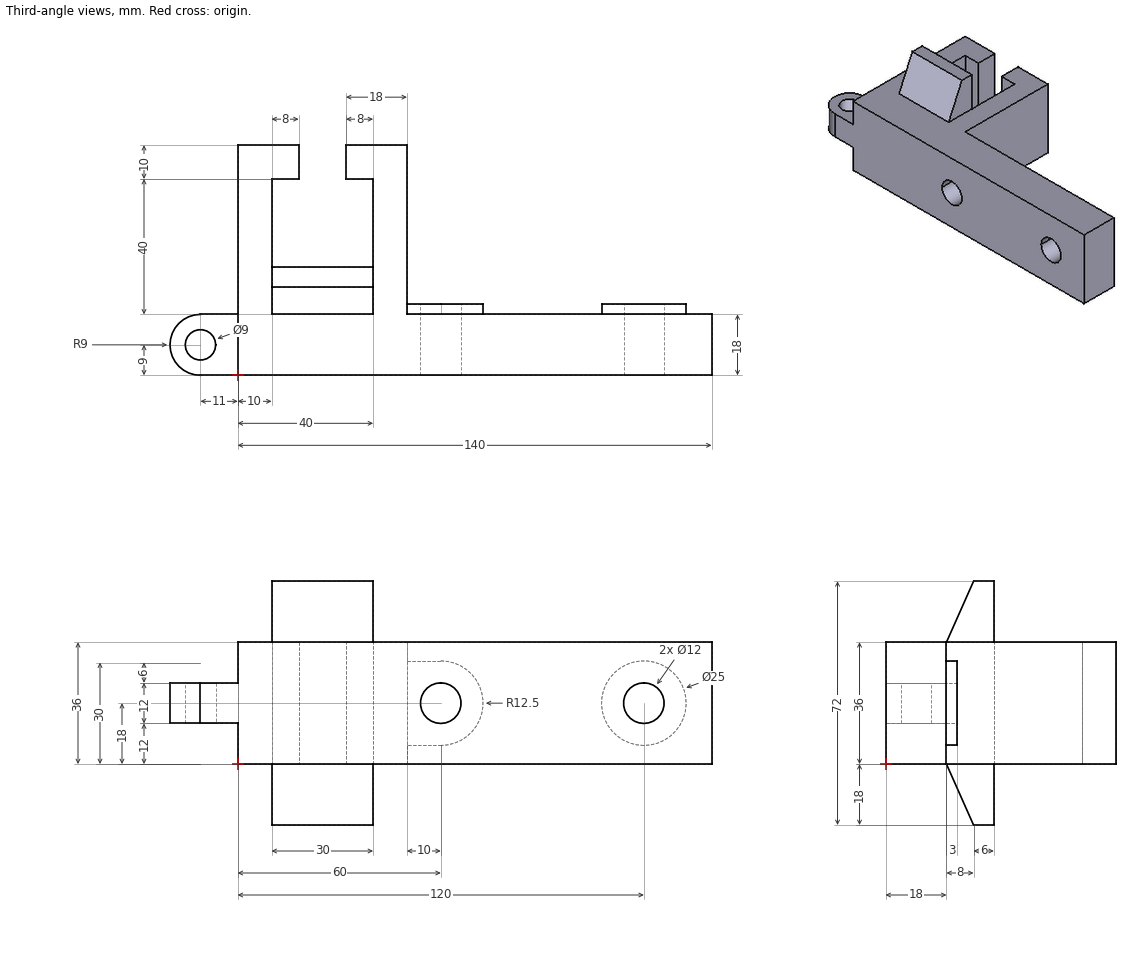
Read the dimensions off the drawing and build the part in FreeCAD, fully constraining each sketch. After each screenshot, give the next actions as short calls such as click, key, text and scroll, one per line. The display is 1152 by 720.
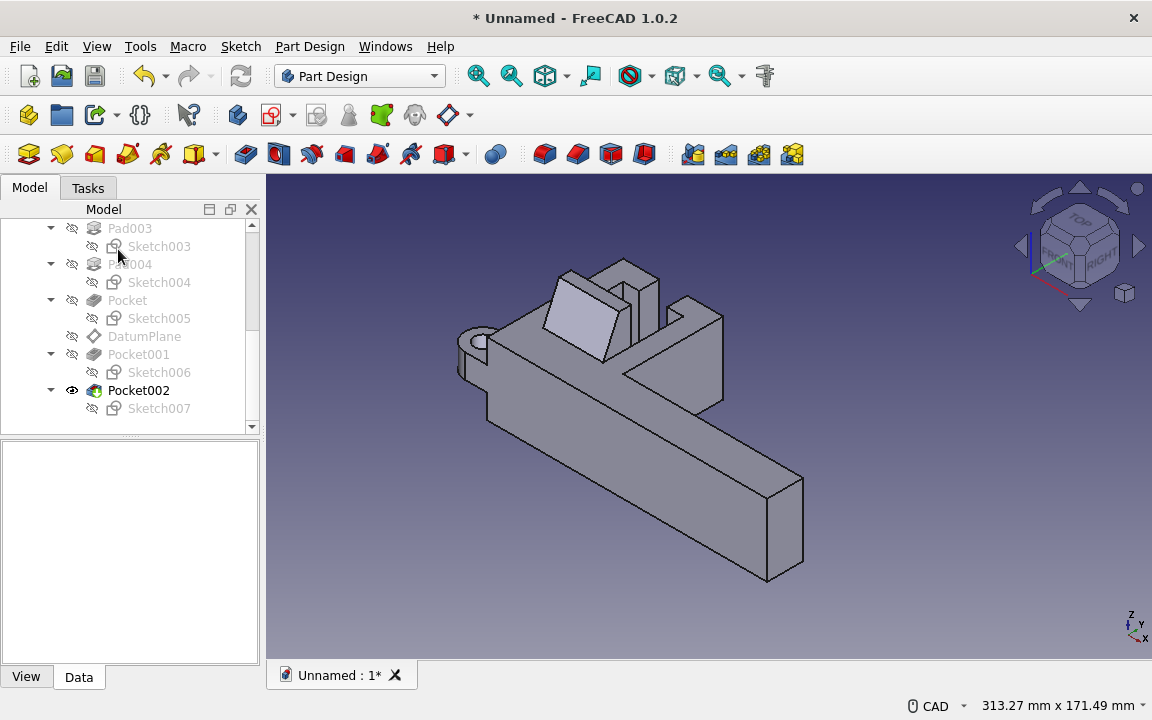
key(4)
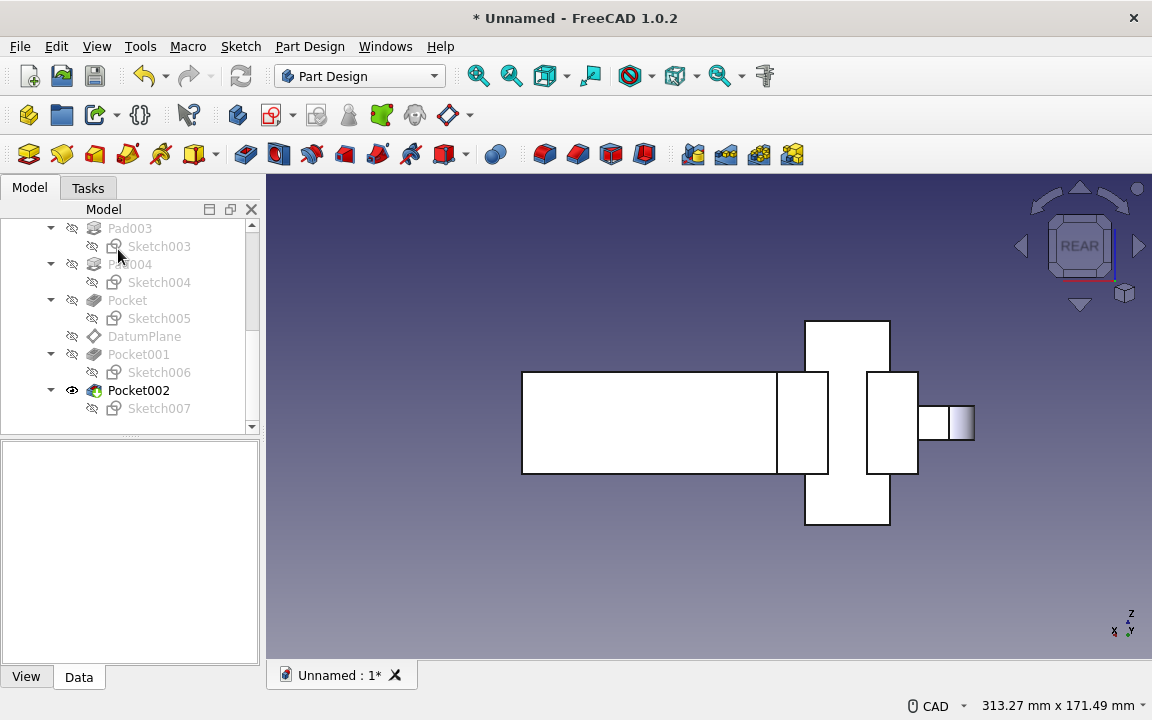
click(577, 422)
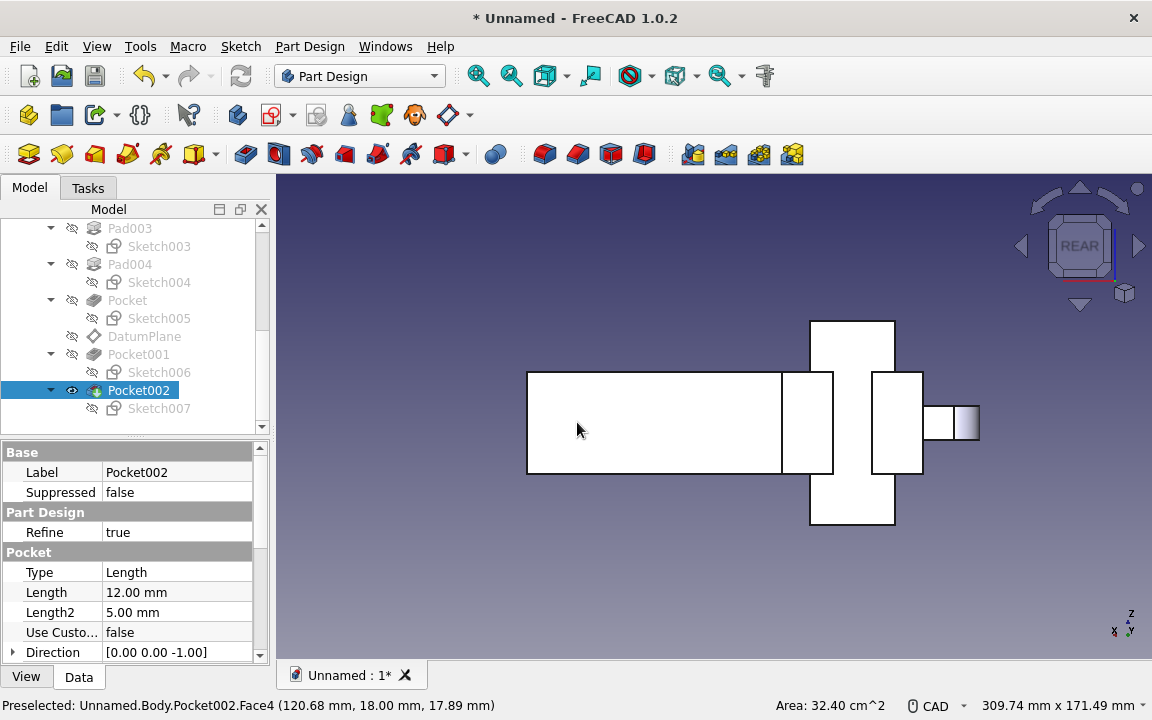
click(270, 116)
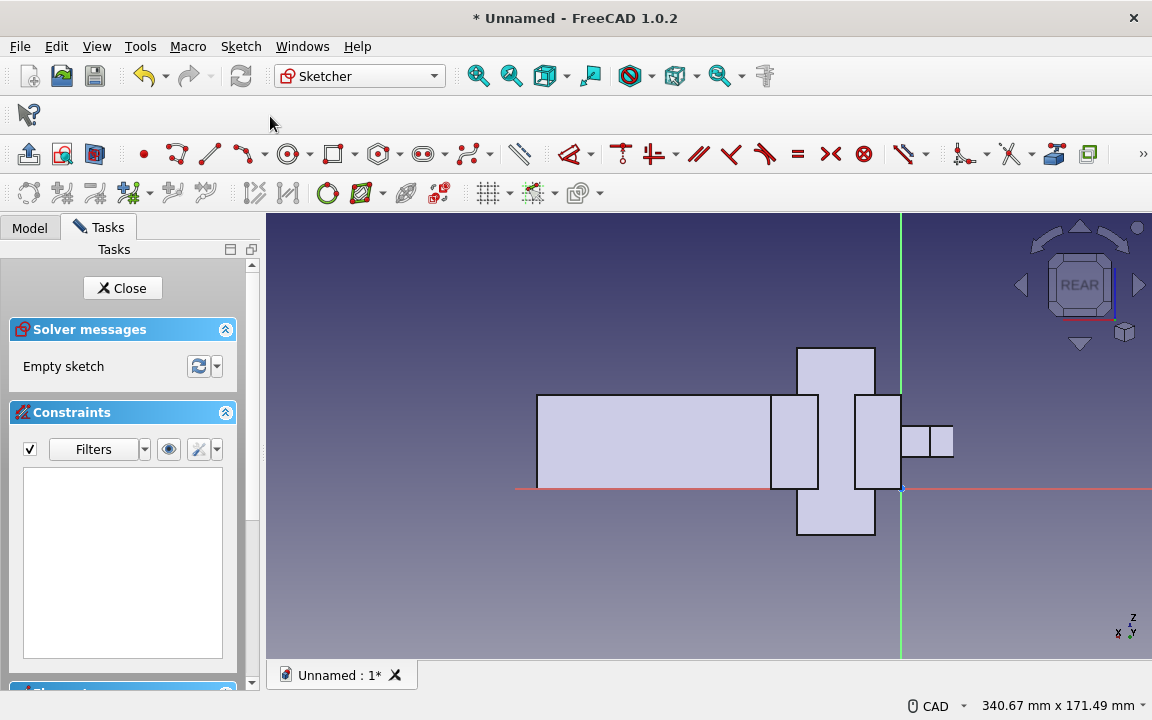
scroll(775, 444, up, 7)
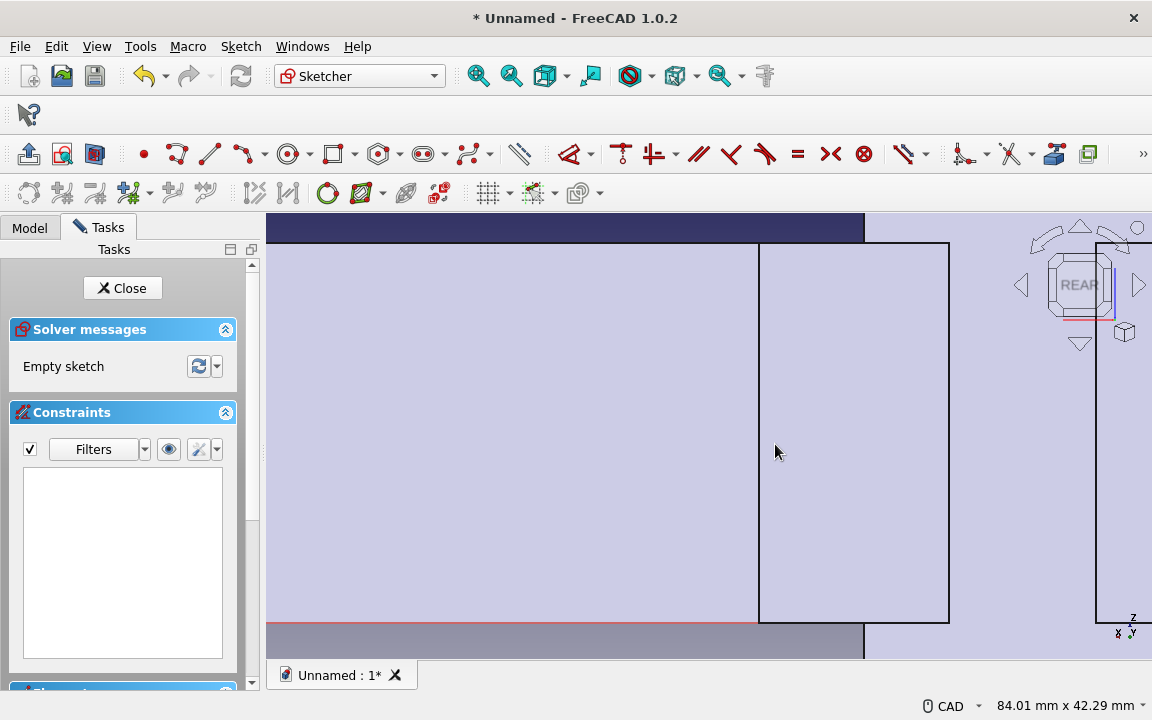
key(g)
key(m)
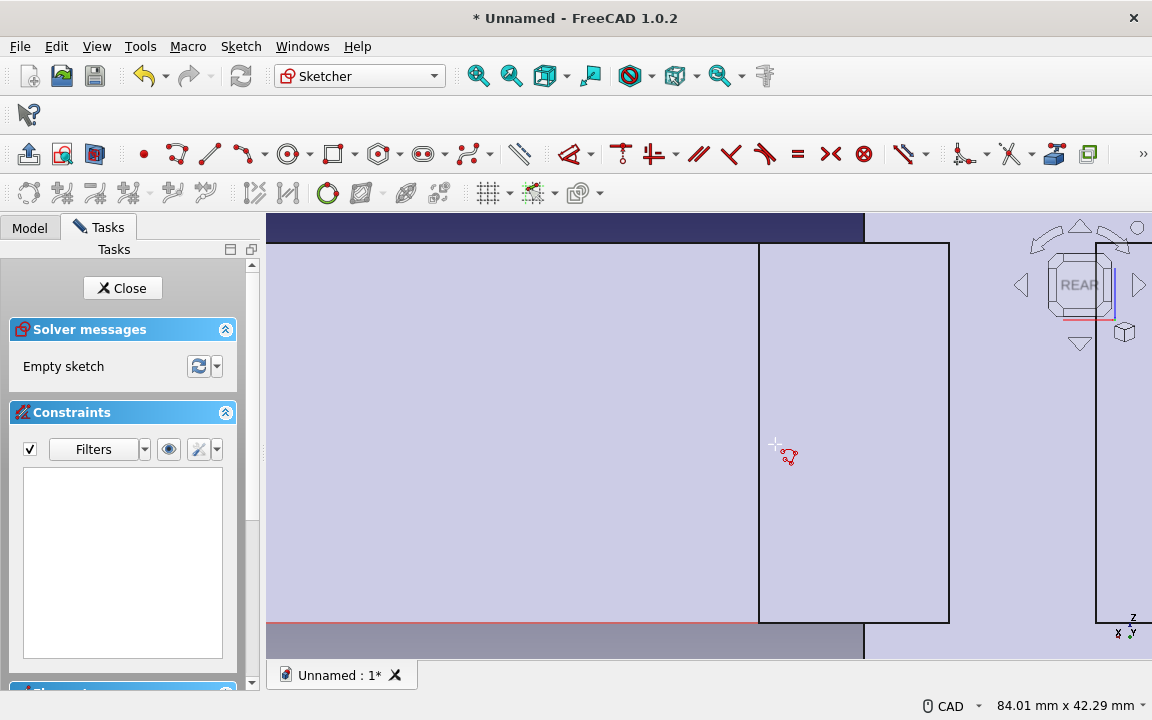
click(653, 565)
click(759, 565)
click(759, 301)
click(653, 301)
right_click(653, 301)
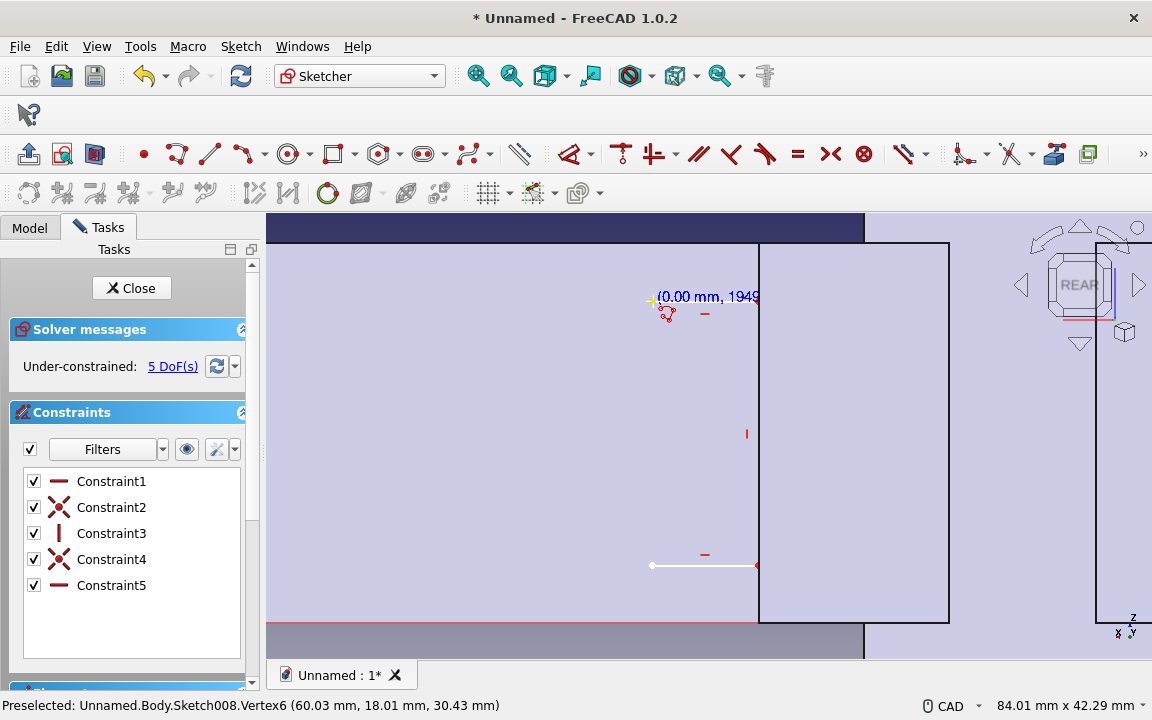
key(g)
key(3)
key(a)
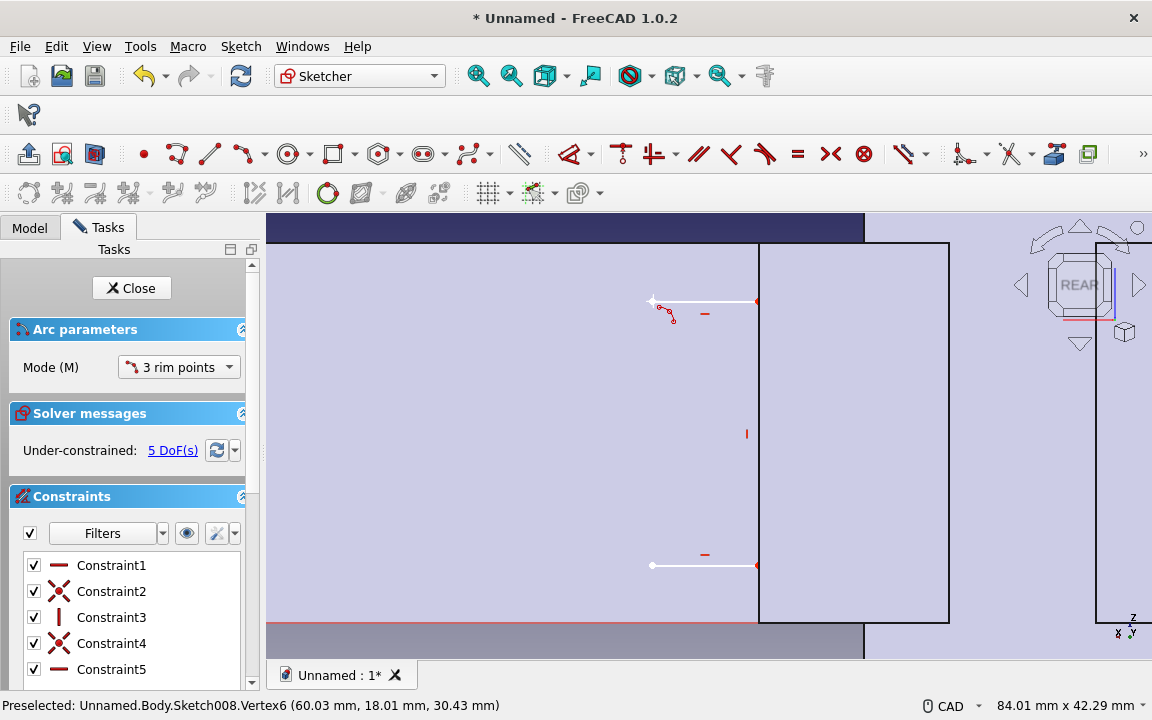
click(653, 302)
click(653, 566)
click(521, 433)
key(Escape)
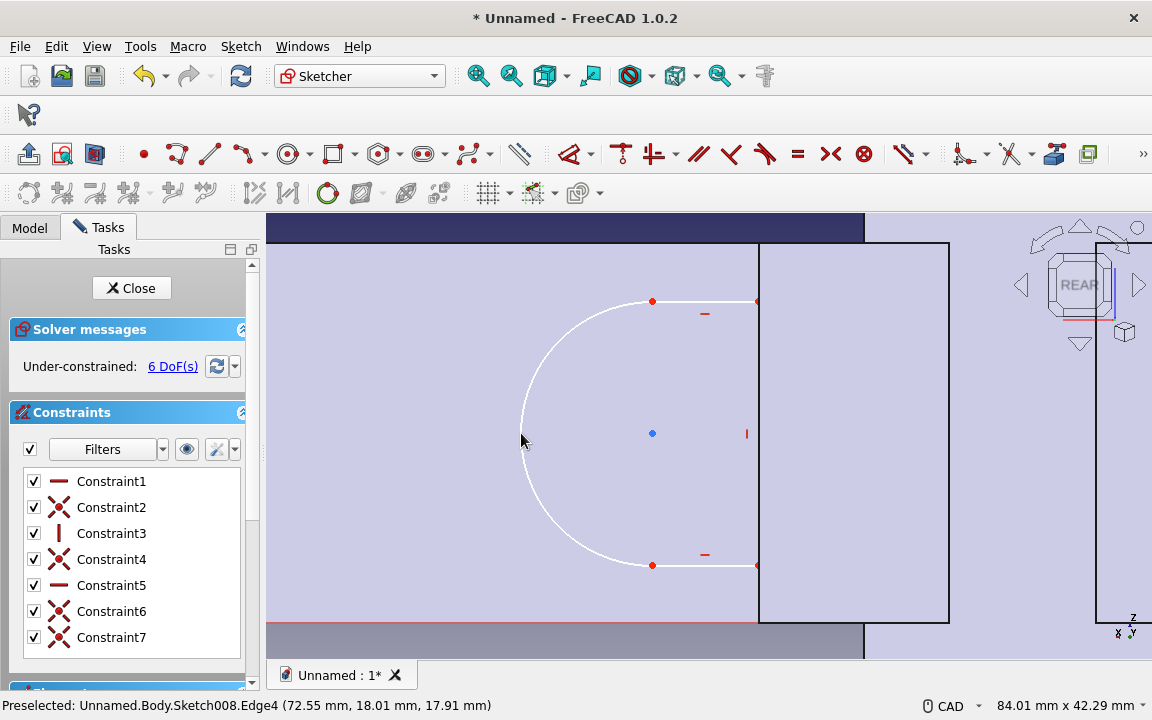
click(685, 566)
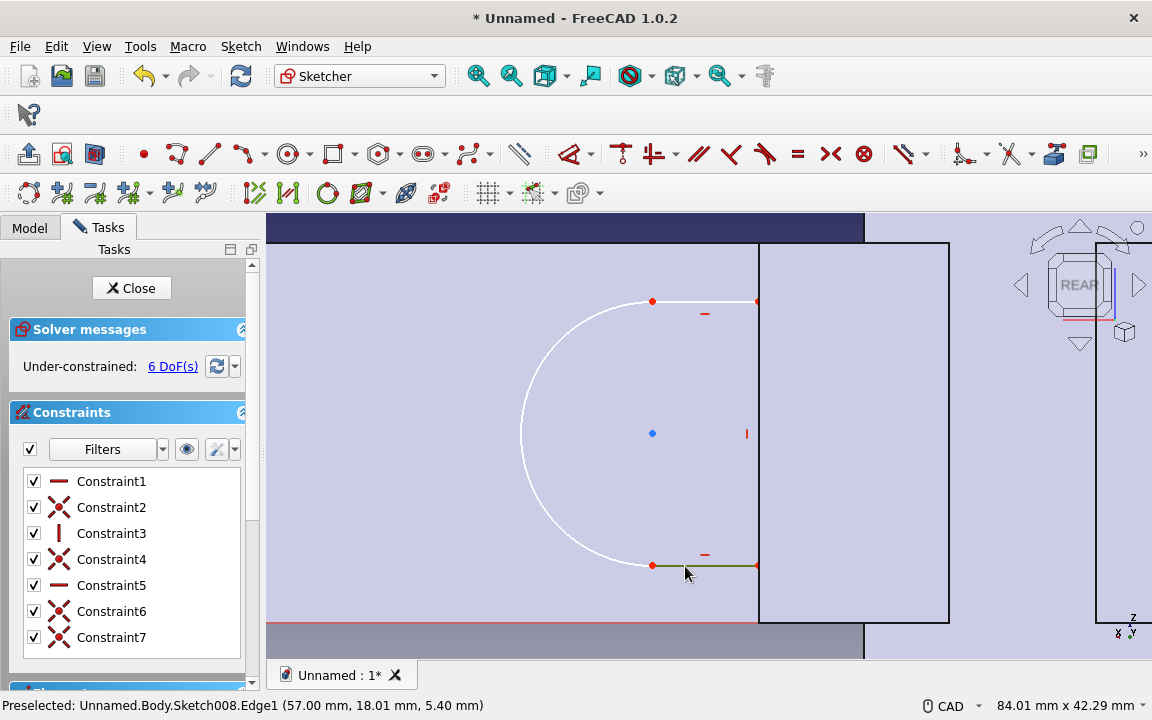
click(546, 356)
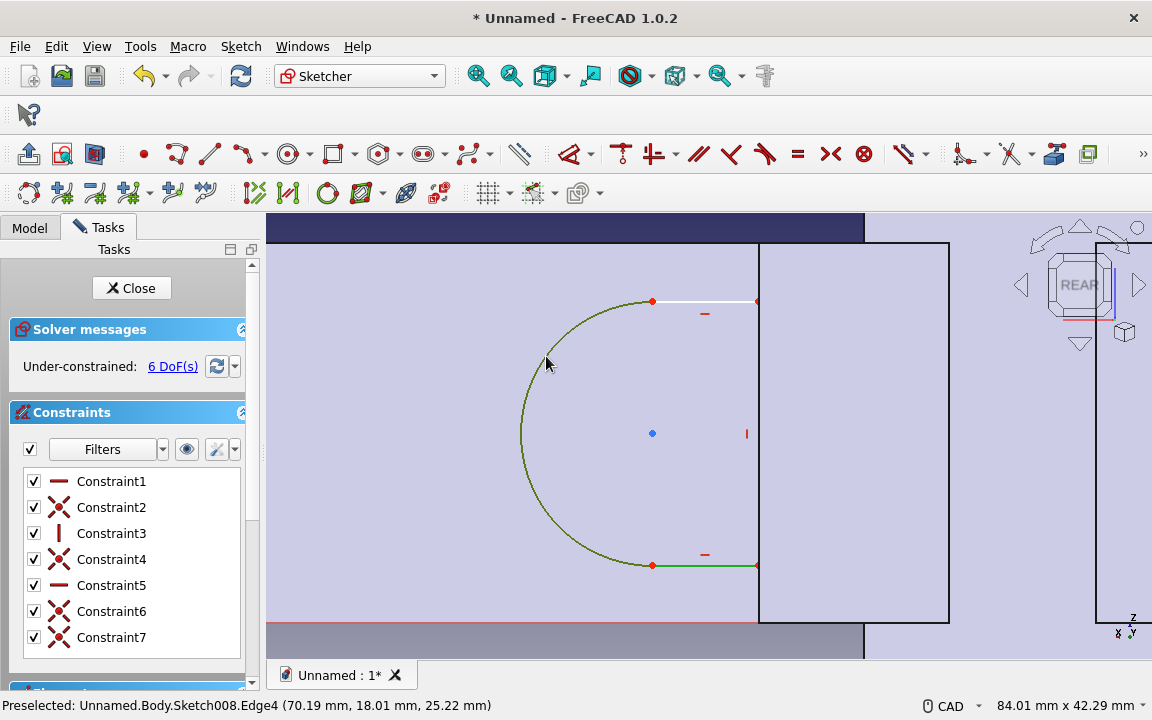
click(765, 154)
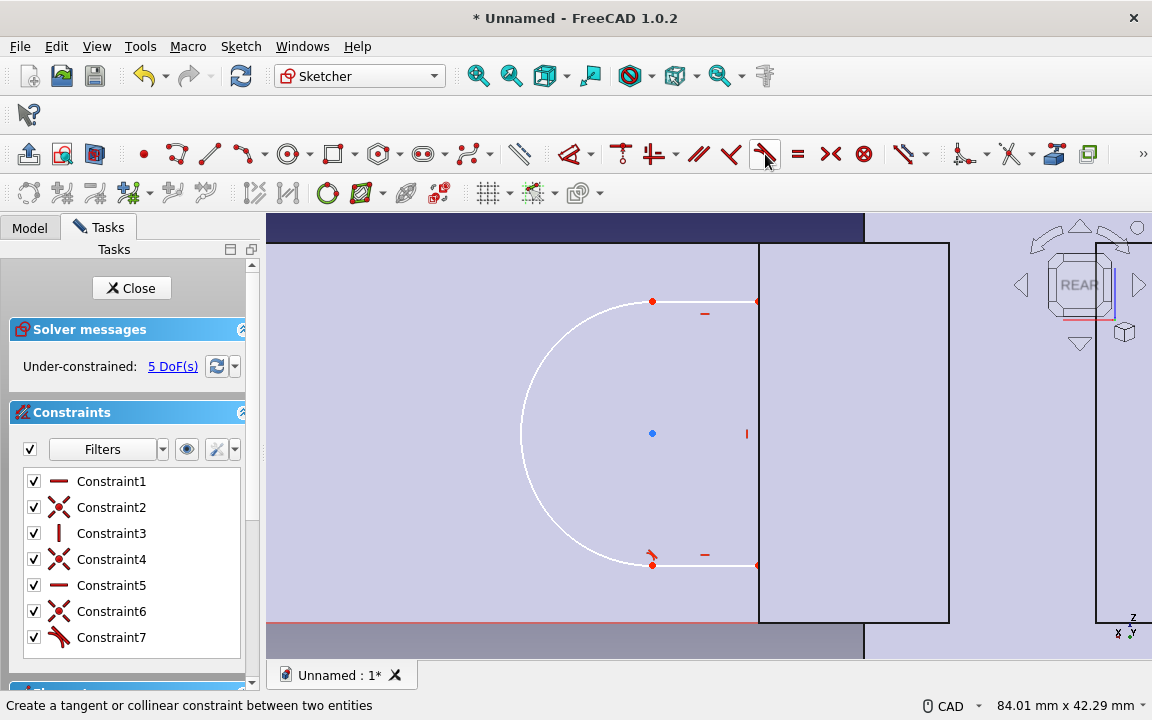
click(727, 302)